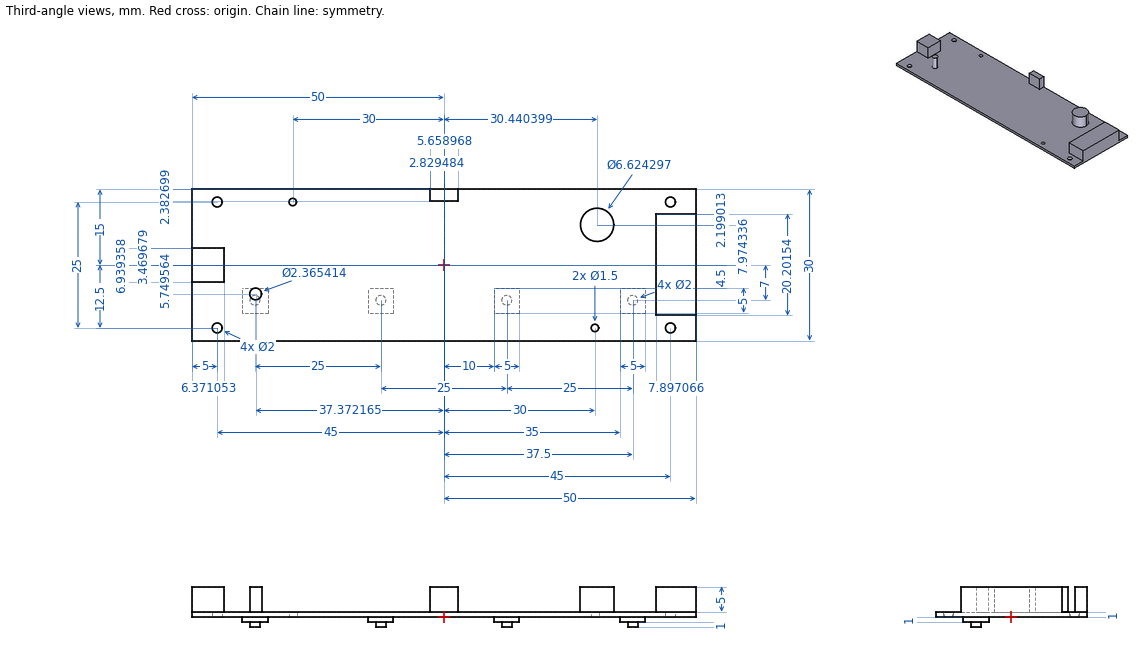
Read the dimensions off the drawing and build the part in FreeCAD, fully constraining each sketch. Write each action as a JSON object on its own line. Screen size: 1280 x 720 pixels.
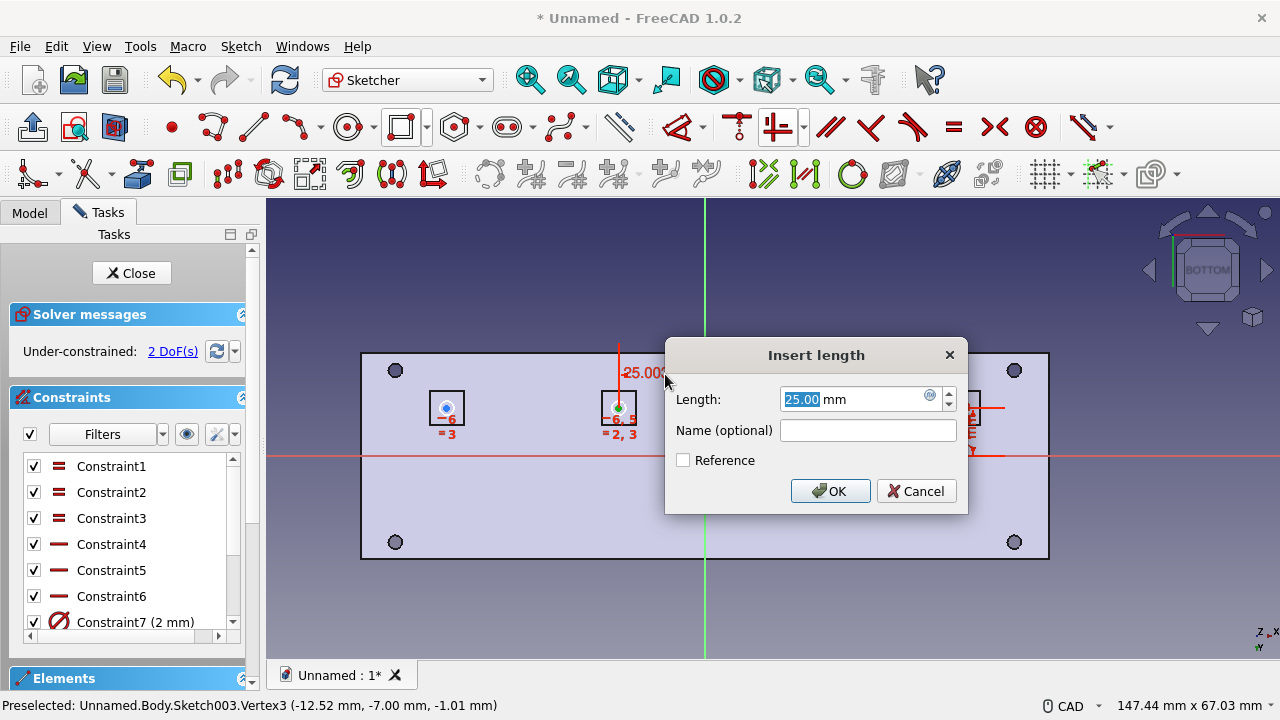
{"action": "type", "text": "25"}
{"action": "key", "text": "Return"}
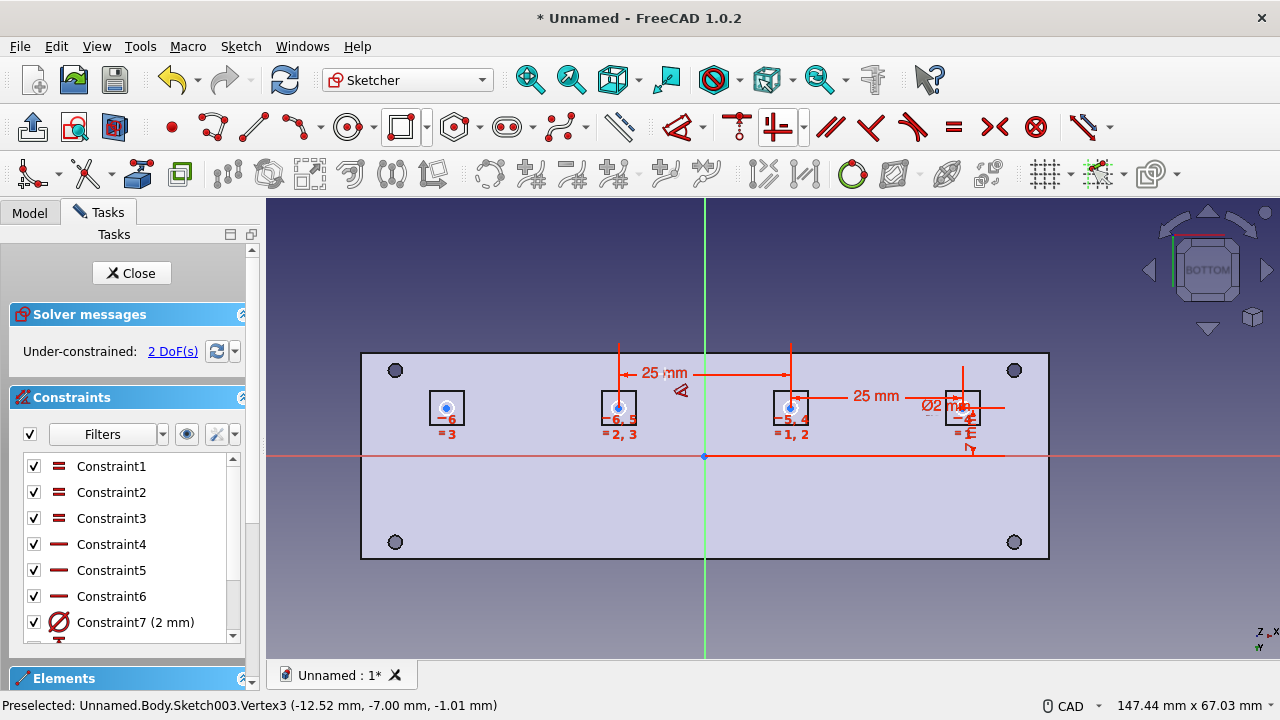
{"action": "left_click", "coordinate": [619, 408]}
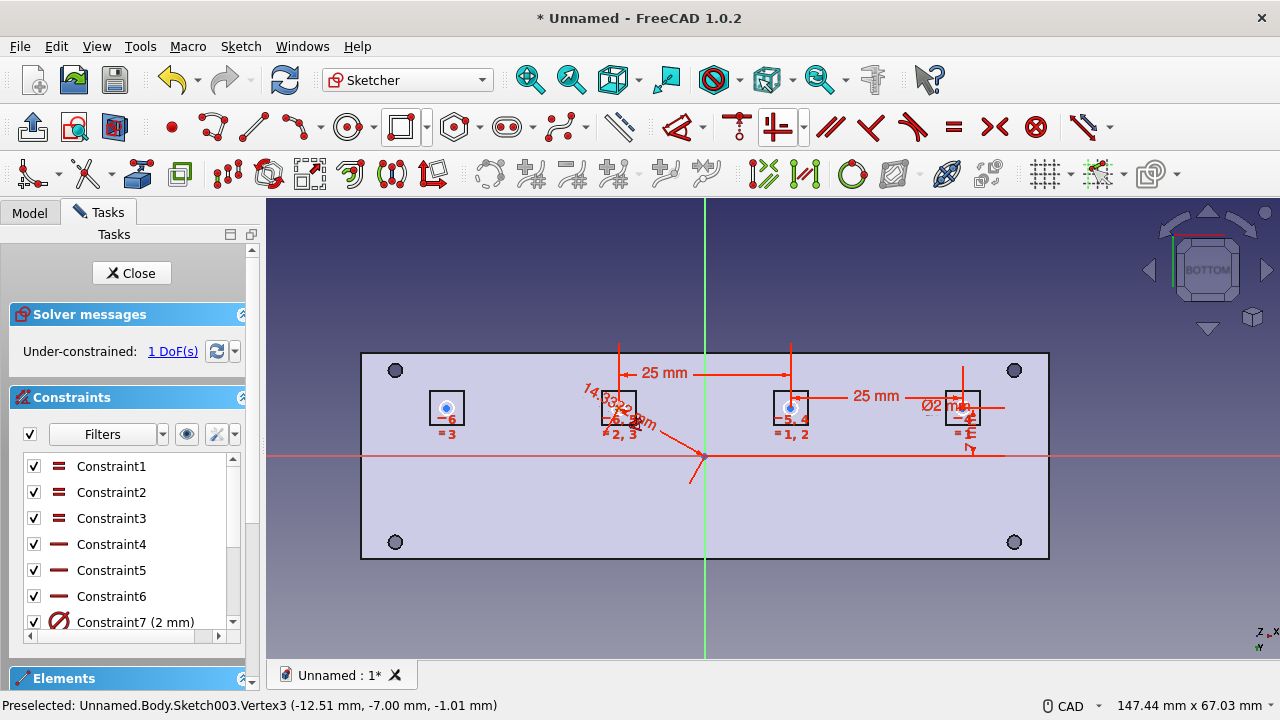
{"action": "left_click", "coordinate": [447, 408]}
{"action": "left_click", "coordinate": [533, 374]}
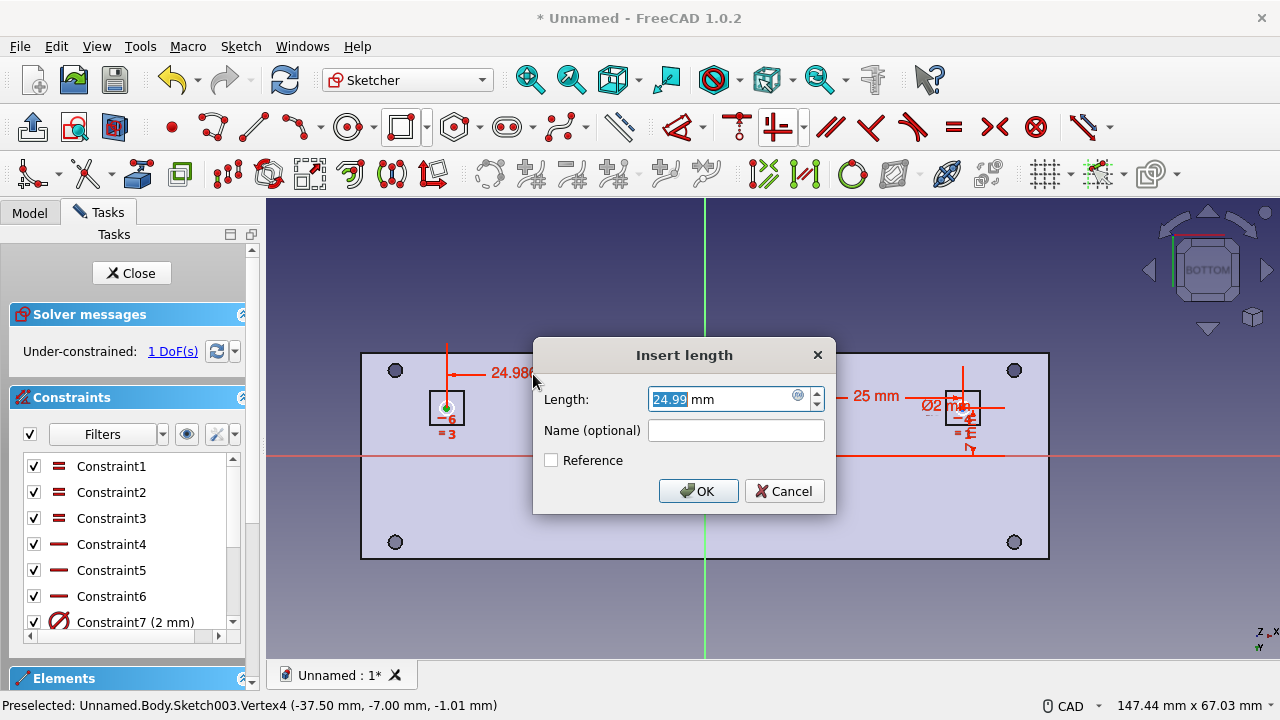
{"action": "type", "text": "25"}
{"action": "key", "text": "Return"}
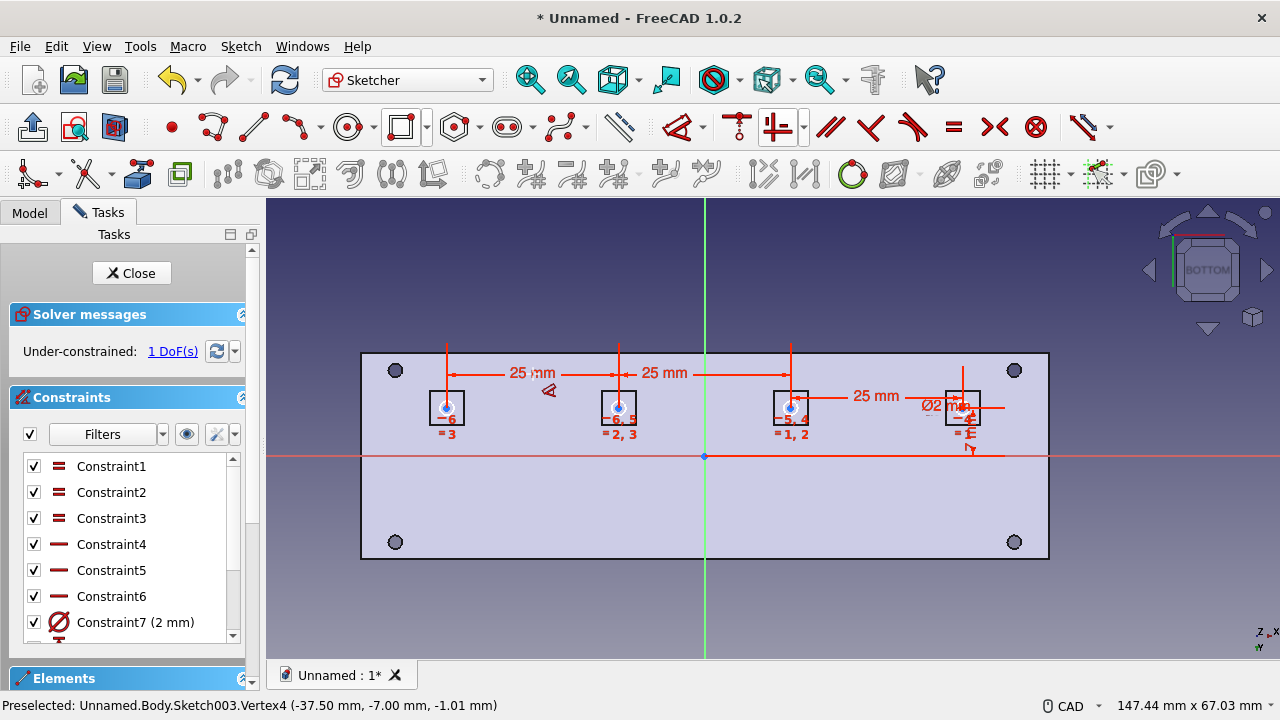
{"action": "left_click", "coordinate": [963, 408]}
{"action": "left_click", "coordinate": [834, 490]}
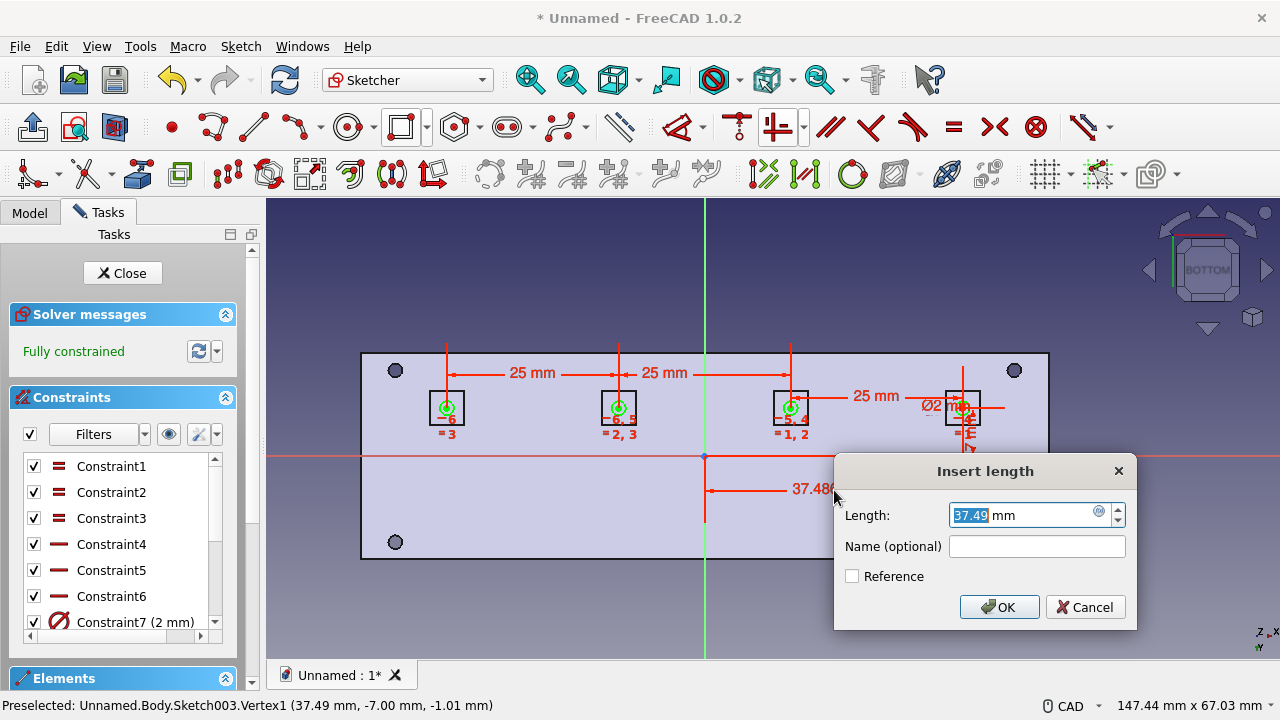
{"action": "type", "text": "37.5"}
{"action": "key", "text": "Return"}
{"action": "key", "text": "Escape"}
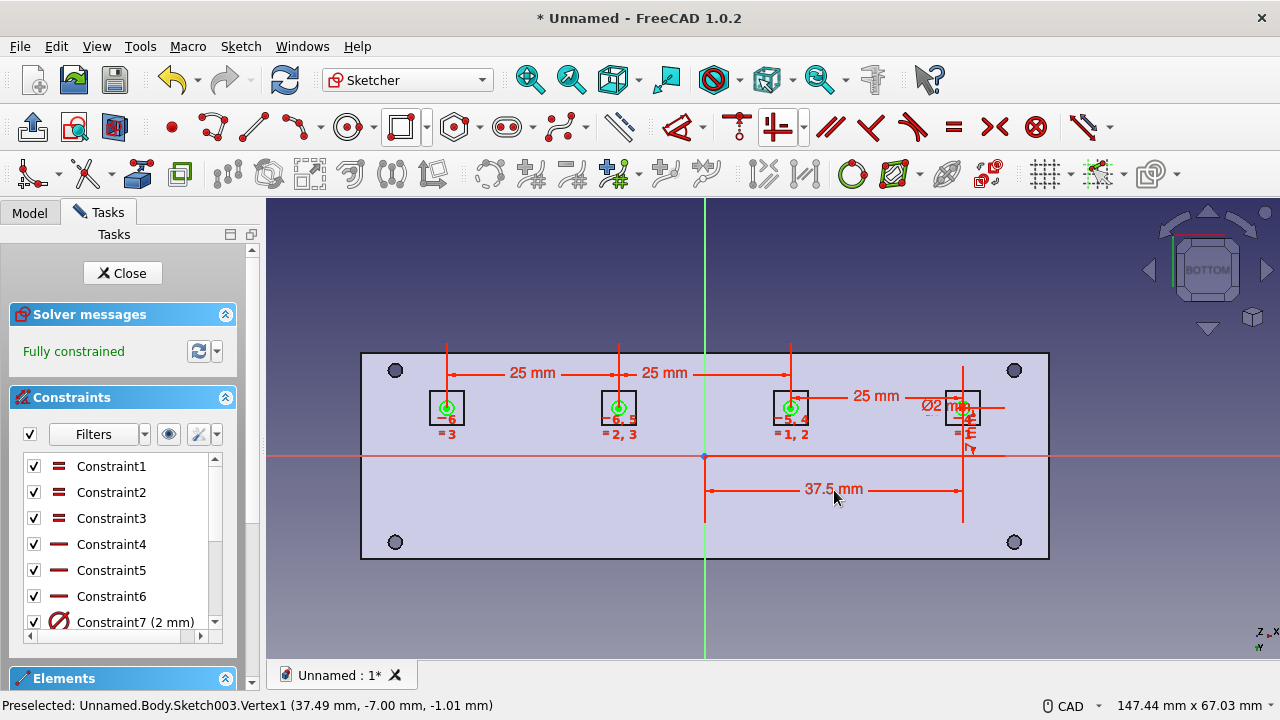
{"action": "left_click", "coordinate": [123, 273]}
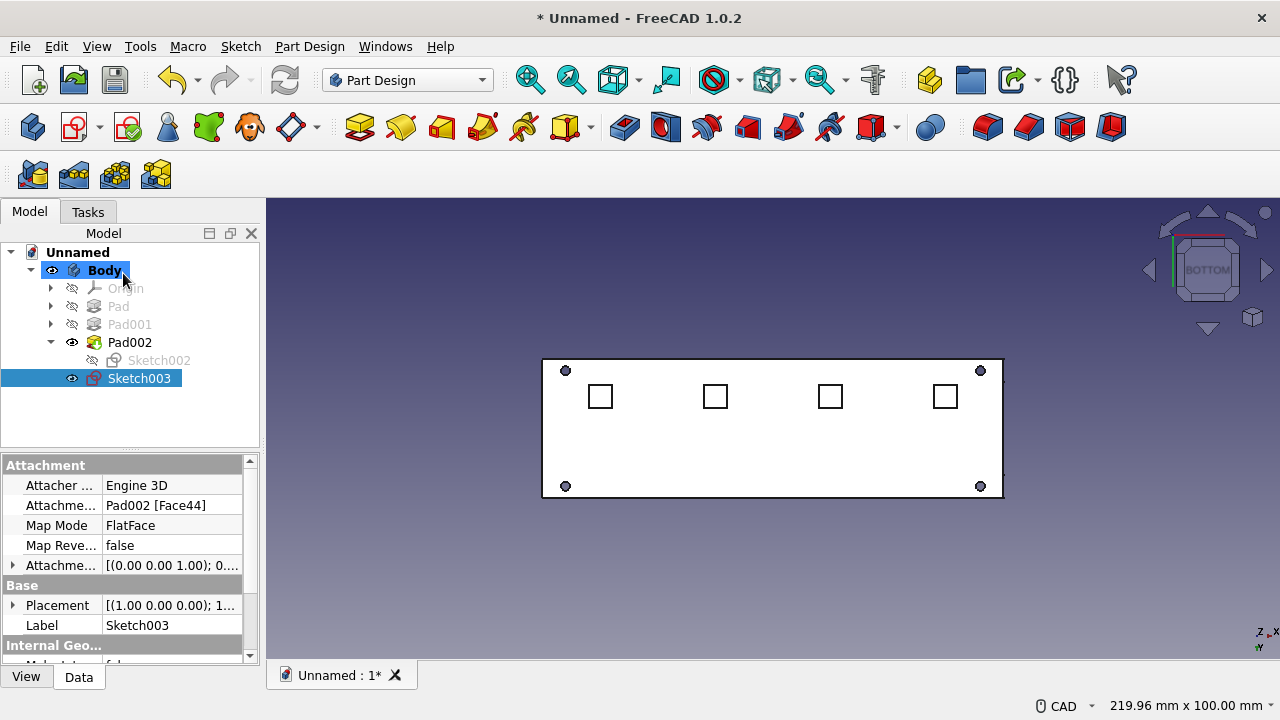
{"action": "left_click", "coordinate": [360, 128]}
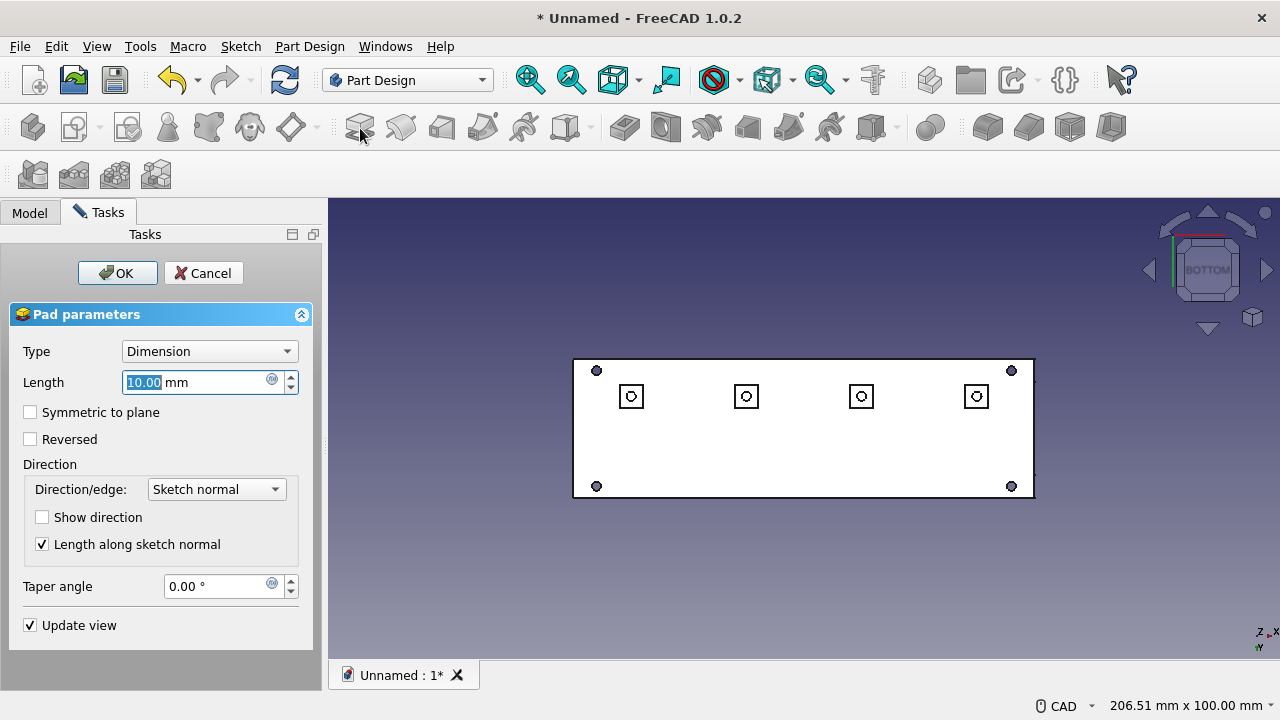
{"action": "type", "text": "1"}
{"action": "key", "text": "Tab"}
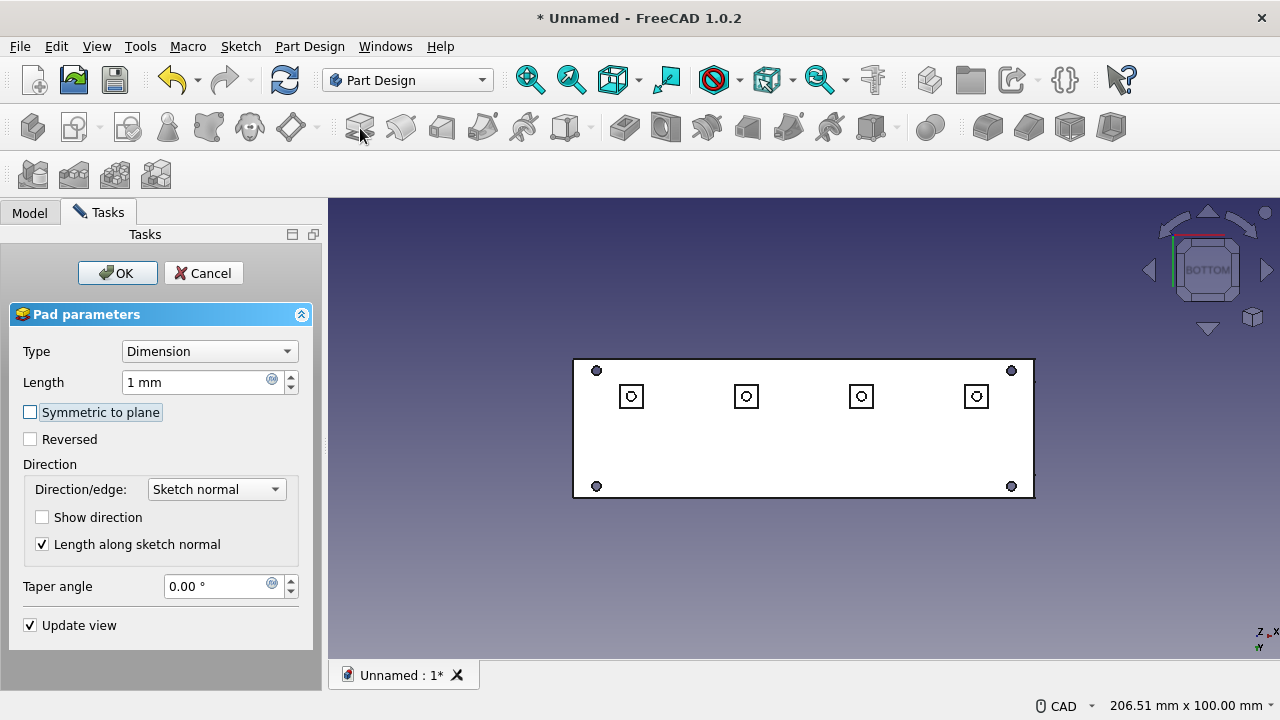
{"action": "left_click", "coordinate": [118, 273]}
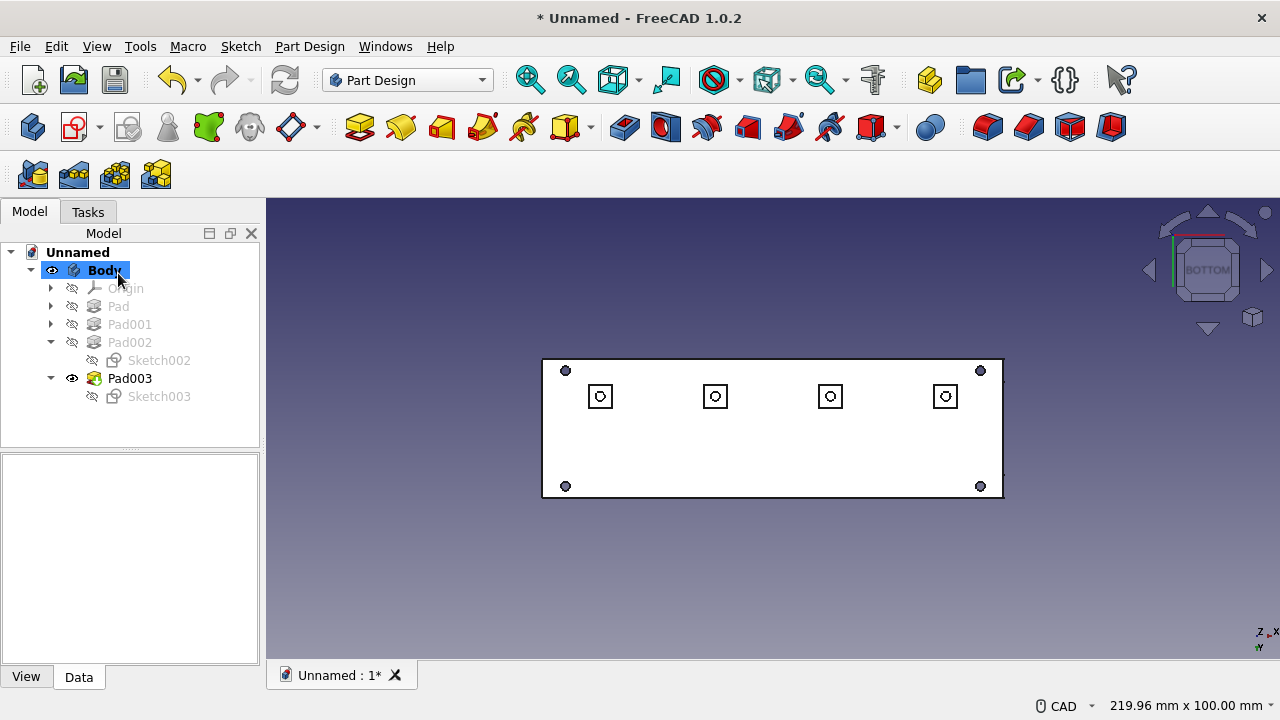
{"action": "key", "text": "0"}